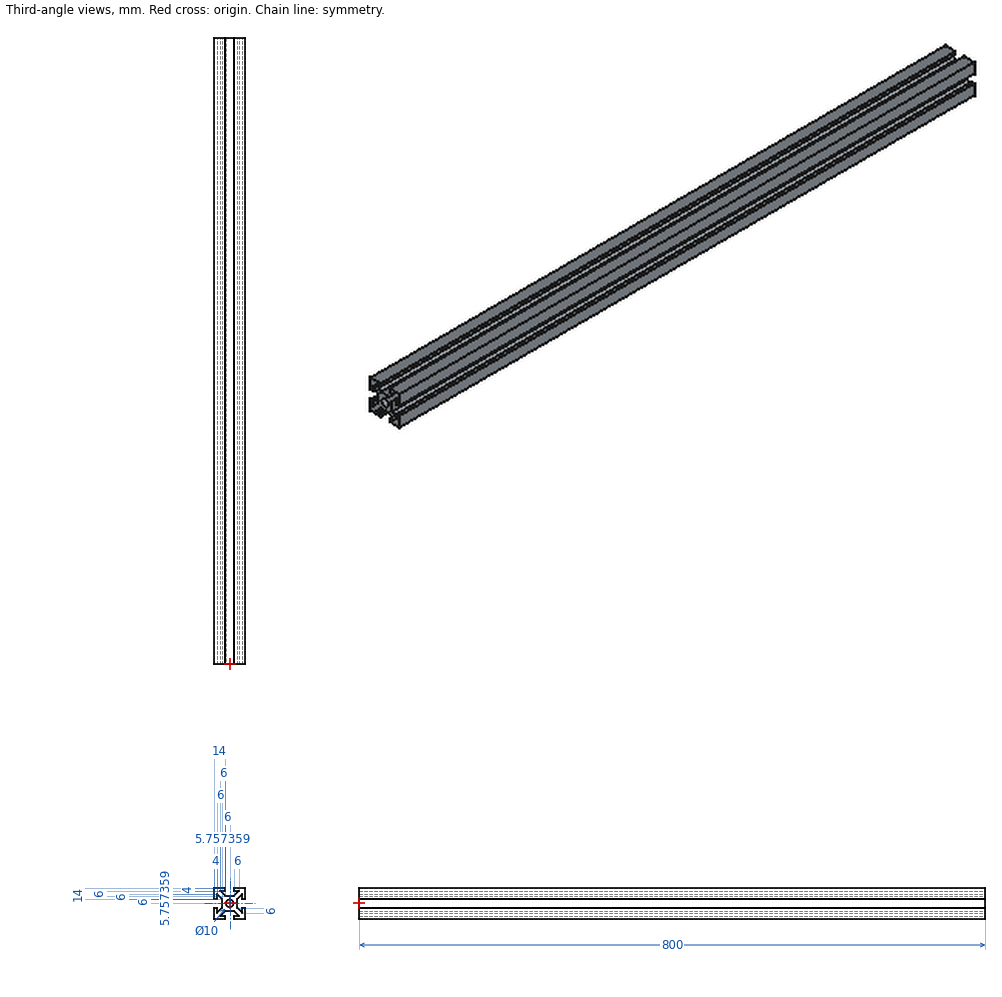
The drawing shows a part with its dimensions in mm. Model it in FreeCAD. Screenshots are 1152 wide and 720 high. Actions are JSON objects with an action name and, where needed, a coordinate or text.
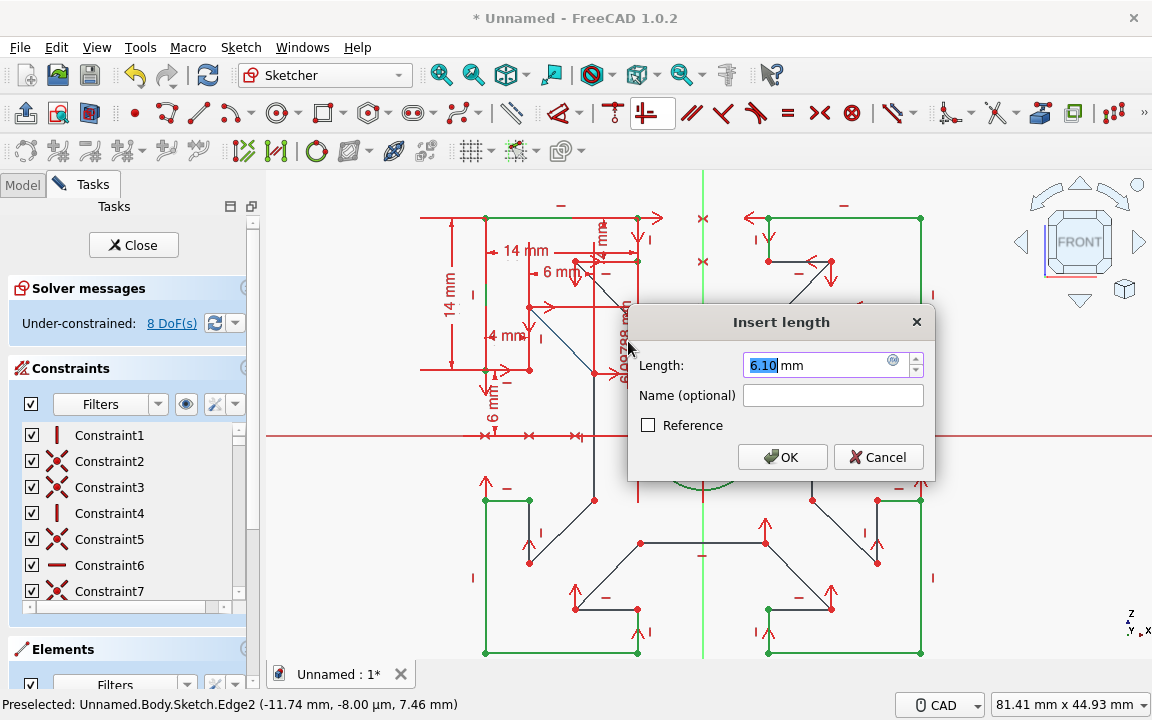
{"action": "type", "text": "6"}
{"action": "key", "text": "Return"}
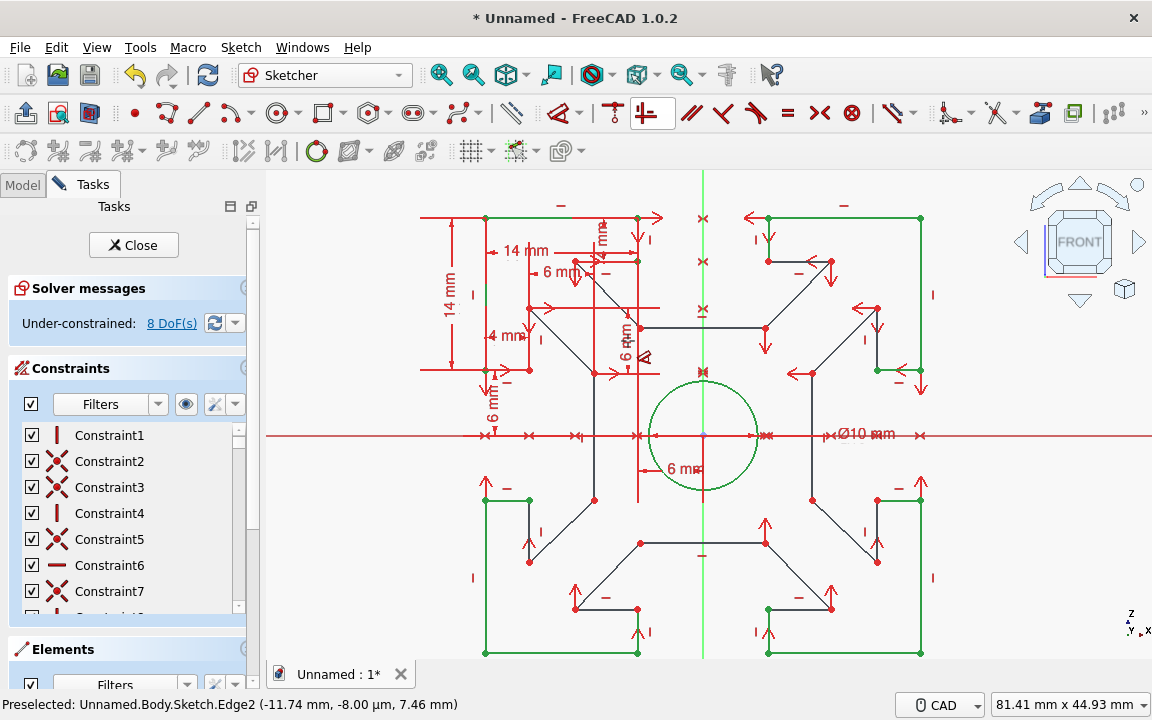
{"action": "left_click", "coordinate": [595, 282]}
{"action": "left_click", "coordinate": [608, 362]}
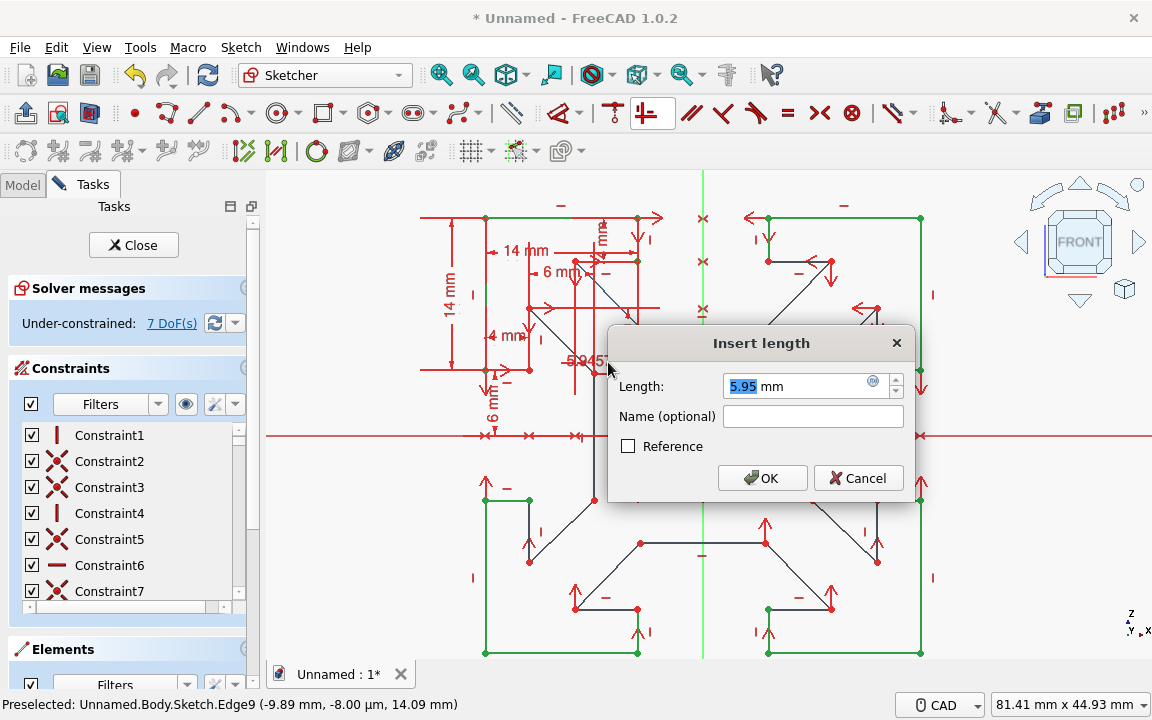
{"action": "type", "text": "6"}
{"action": "key", "text": "Return"}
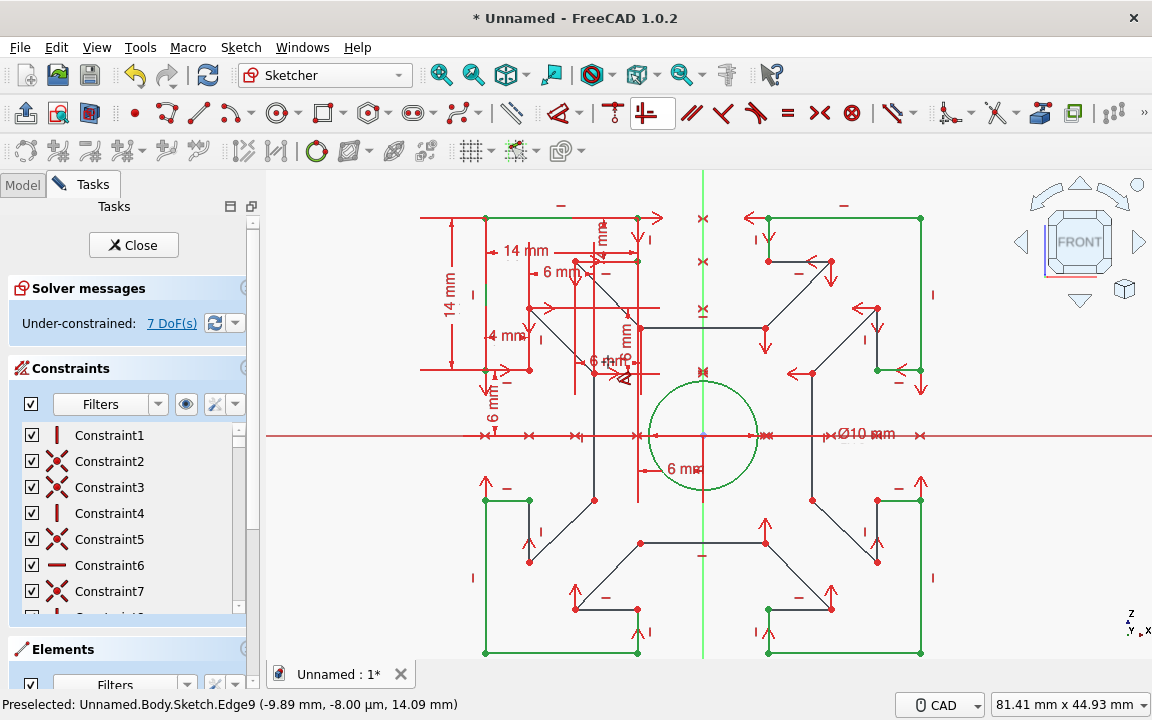
{"action": "left_click", "coordinate": [595, 282]}
{"action": "left_click", "coordinate": [541, 295]}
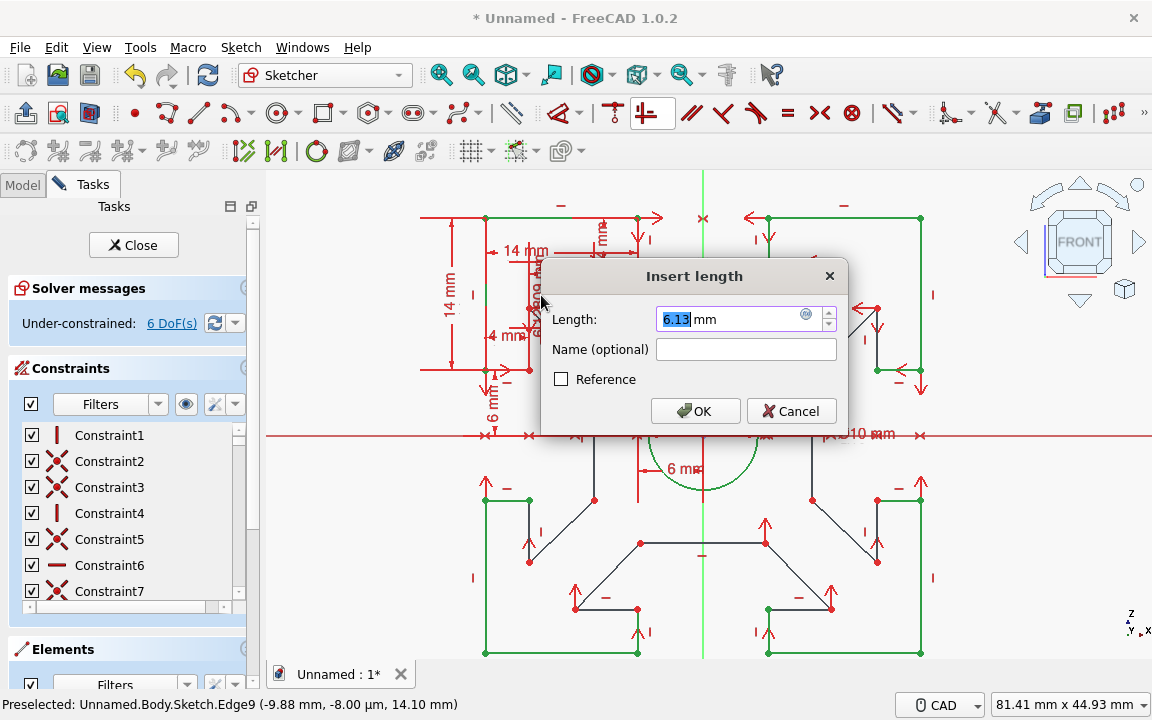
{"action": "type", "text": "6"}
{"action": "key", "text": "Return"}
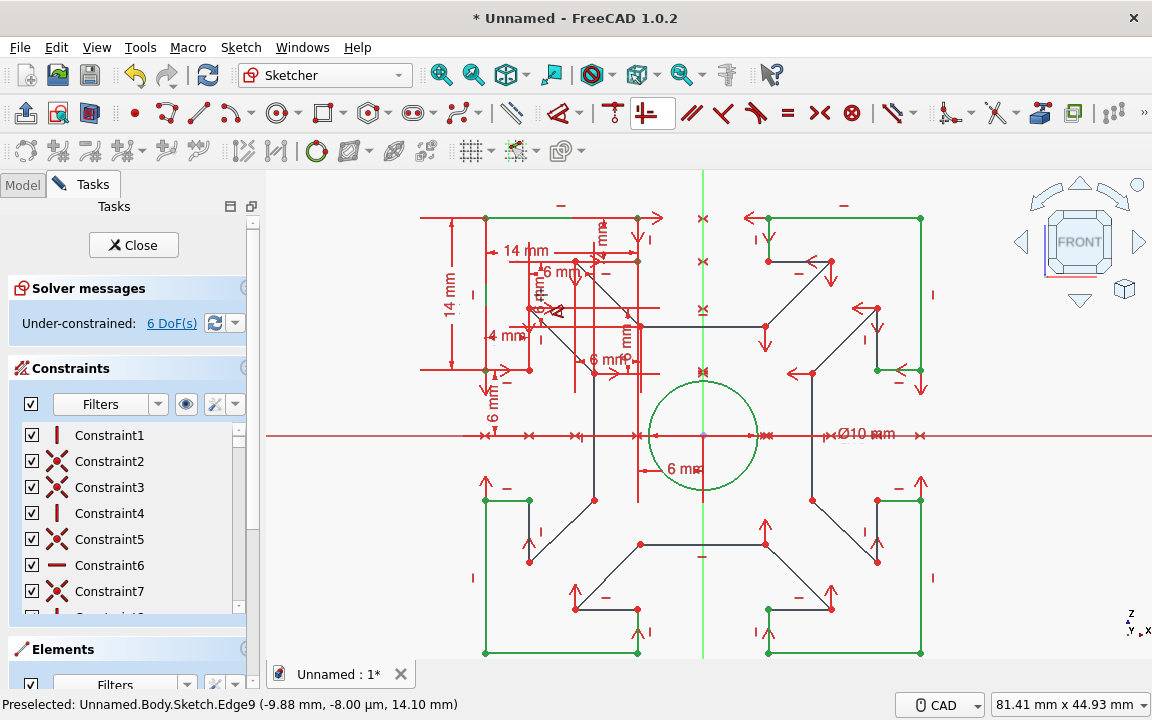
{"action": "left_click", "coordinate": [785, 307]}
{"action": "left_click", "coordinate": [798, 361]}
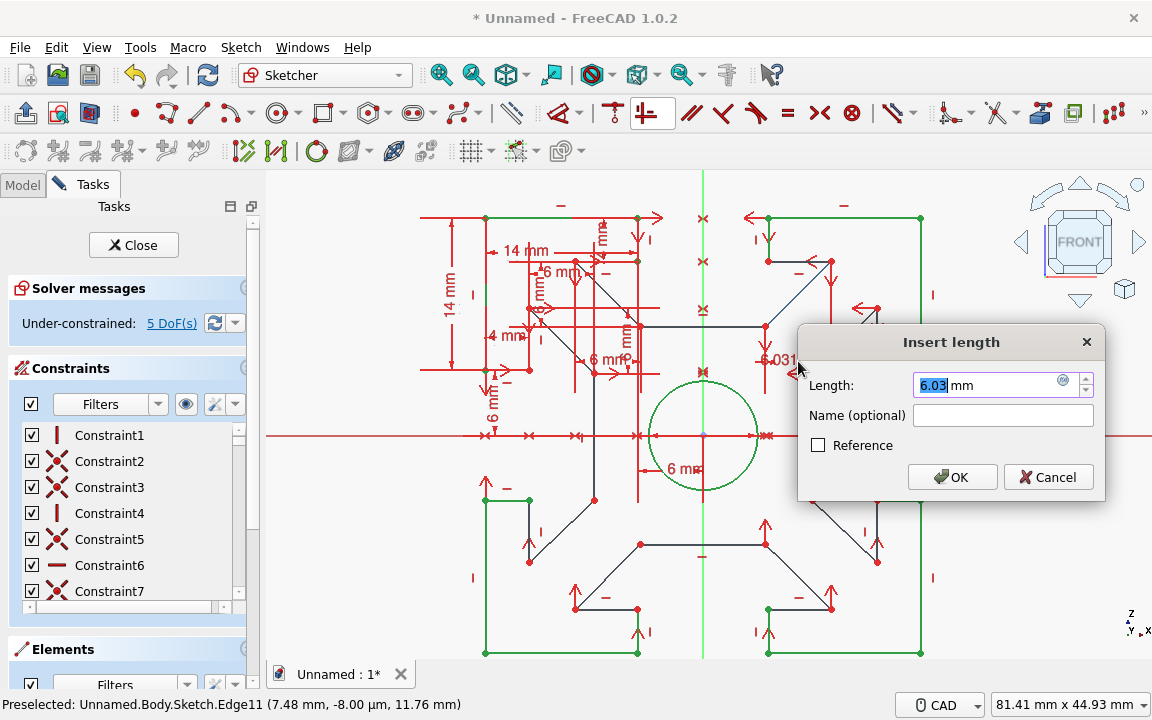
{"action": "type", "text": "6"}
{"action": "key", "text": "Return"}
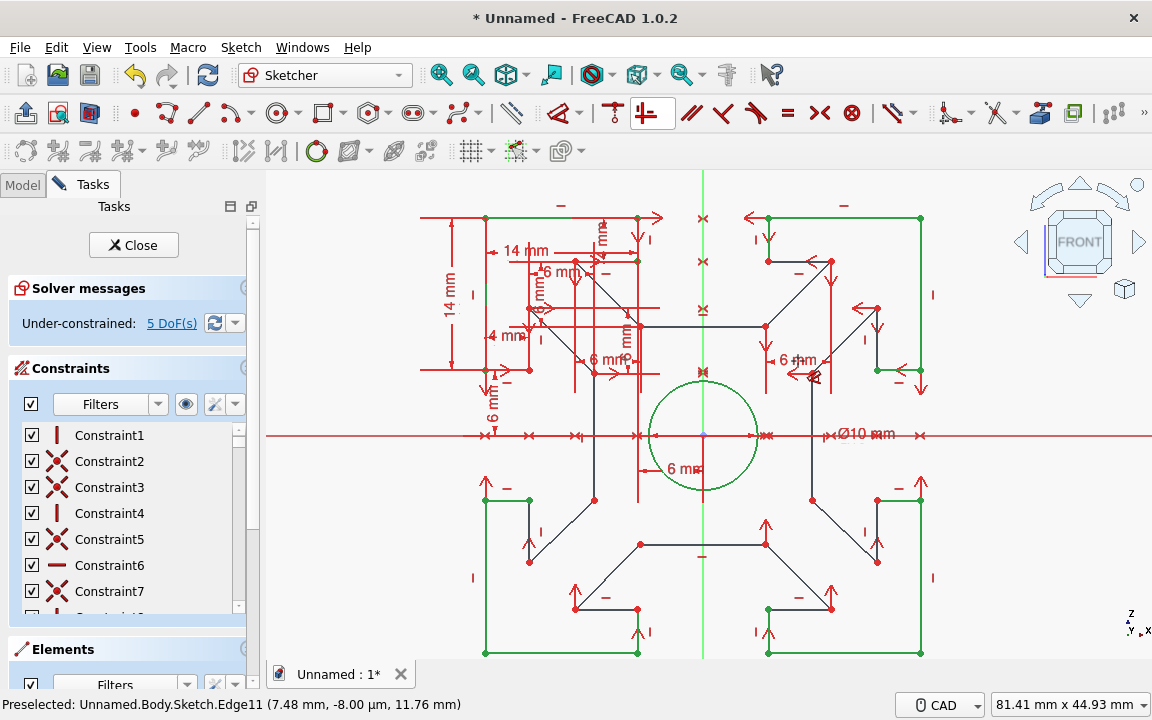
{"action": "left_click", "coordinate": [832, 519]}
{"action": "left_click", "coordinate": [778, 532]}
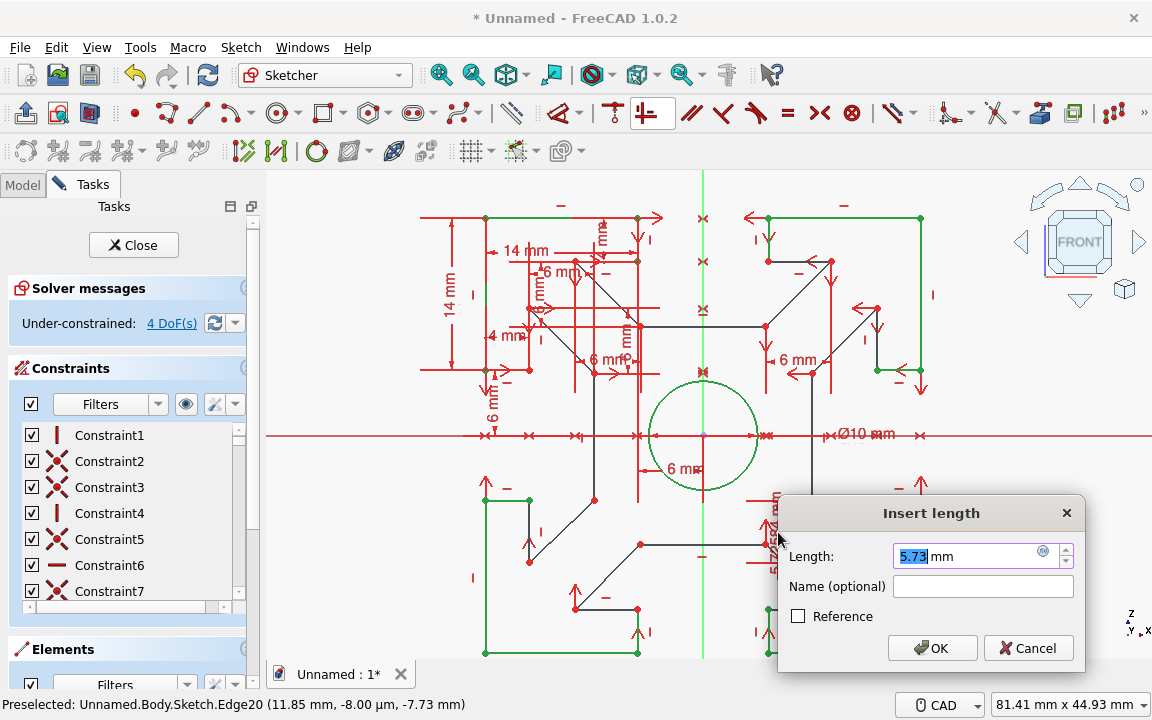
{"action": "type", "text": "6"}
{"action": "key", "text": "Return"}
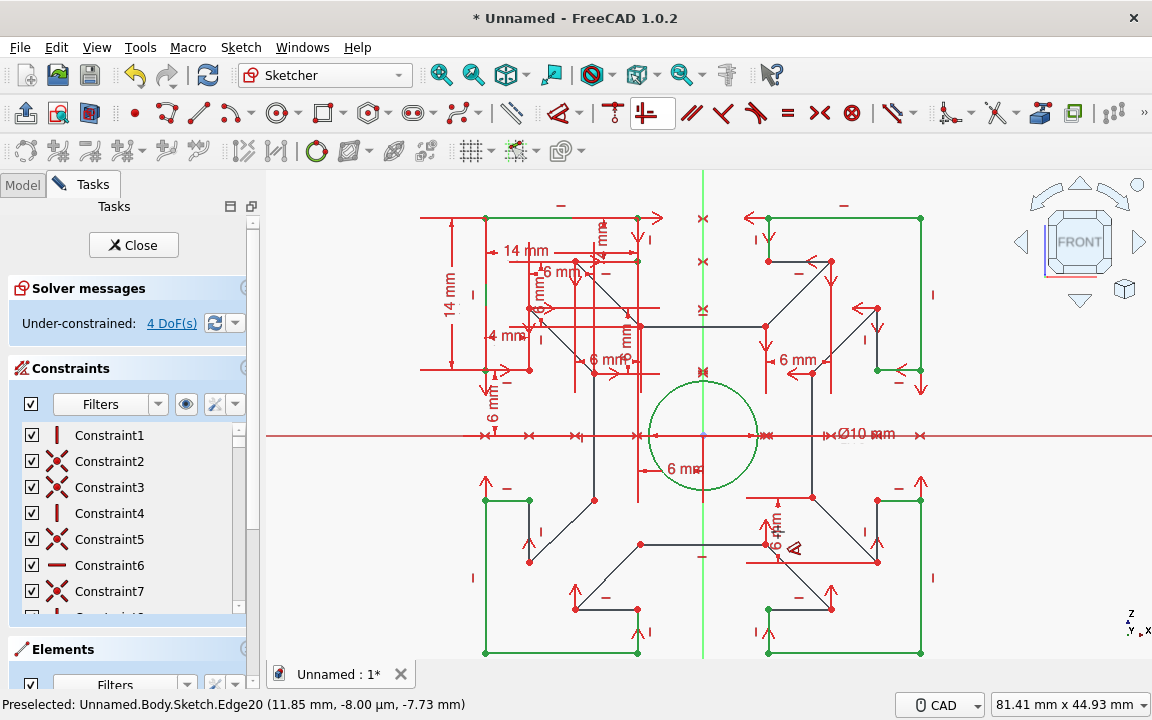
{"action": "left_click", "coordinate": [621, 564]}
{"action": "left_click", "coordinate": [608, 511]}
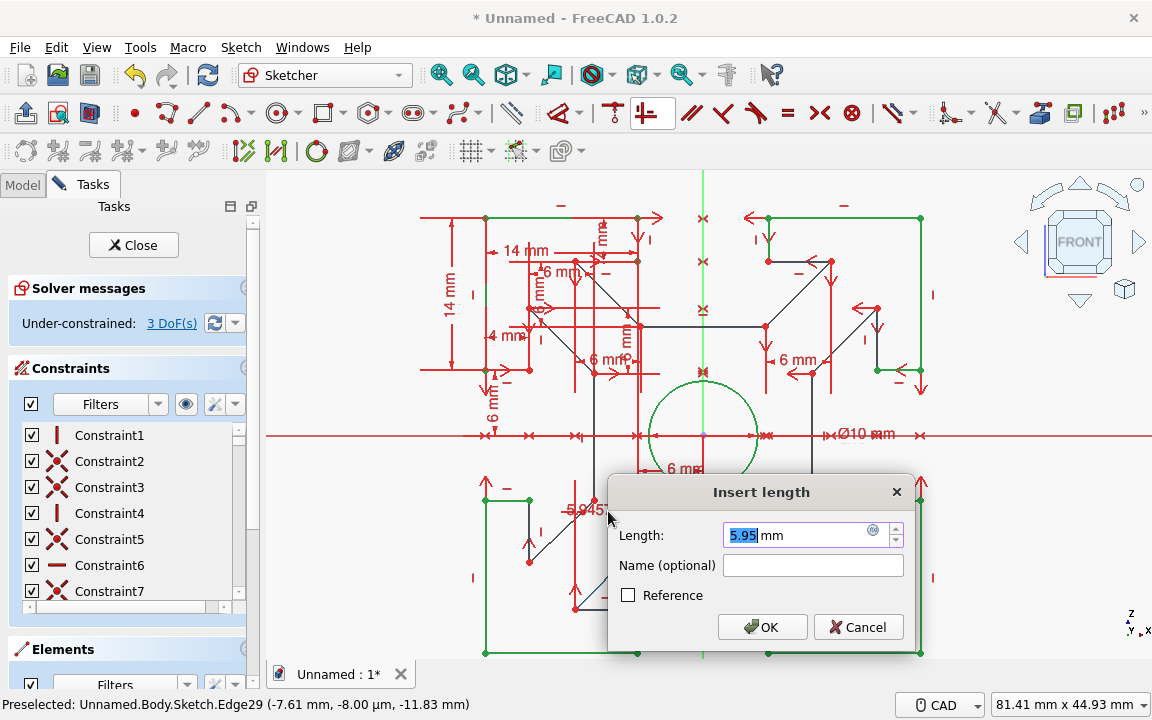
{"action": "type", "text": "6"}
{"action": "key", "text": "Return"}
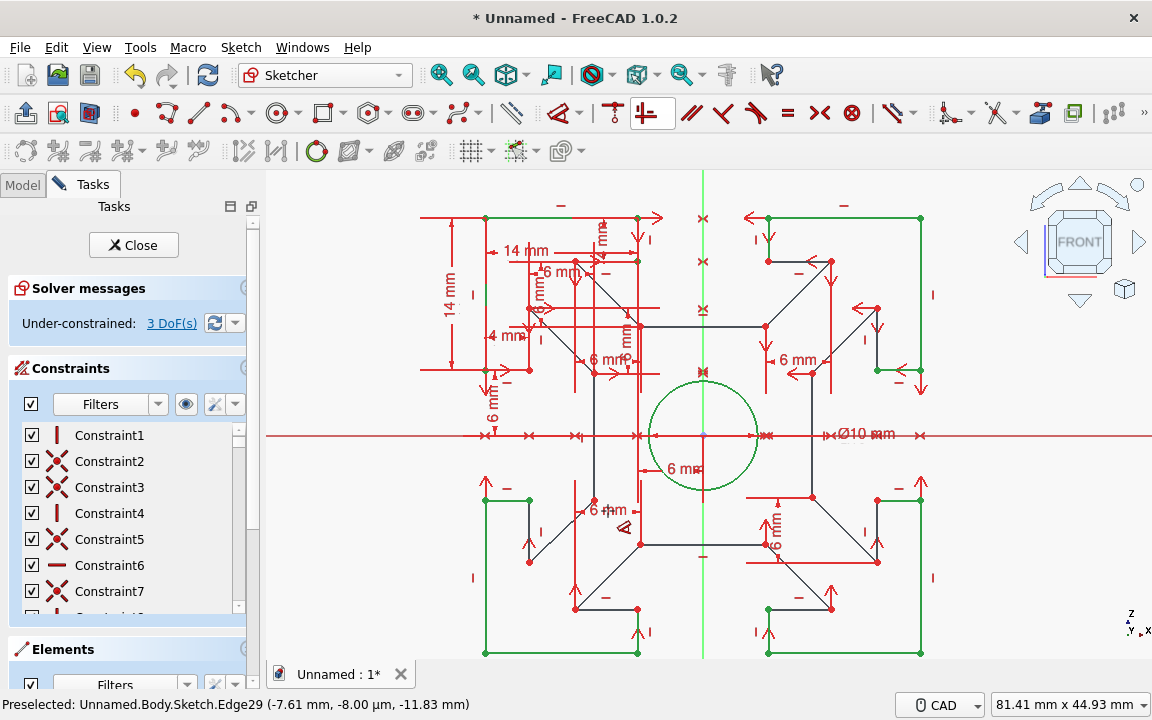
{"action": "left_click", "coordinate": [549, 544]}
{"action": "left_click", "coordinate": [628, 532]}